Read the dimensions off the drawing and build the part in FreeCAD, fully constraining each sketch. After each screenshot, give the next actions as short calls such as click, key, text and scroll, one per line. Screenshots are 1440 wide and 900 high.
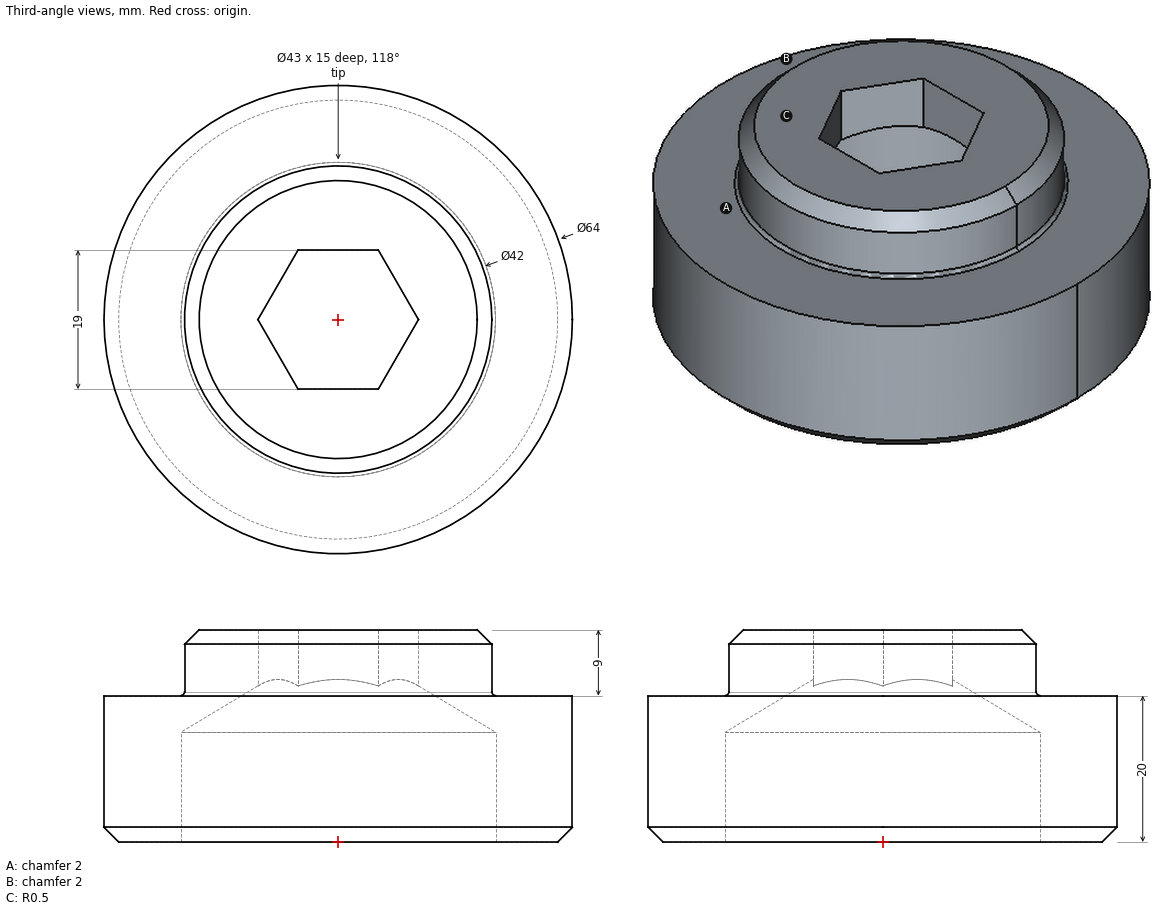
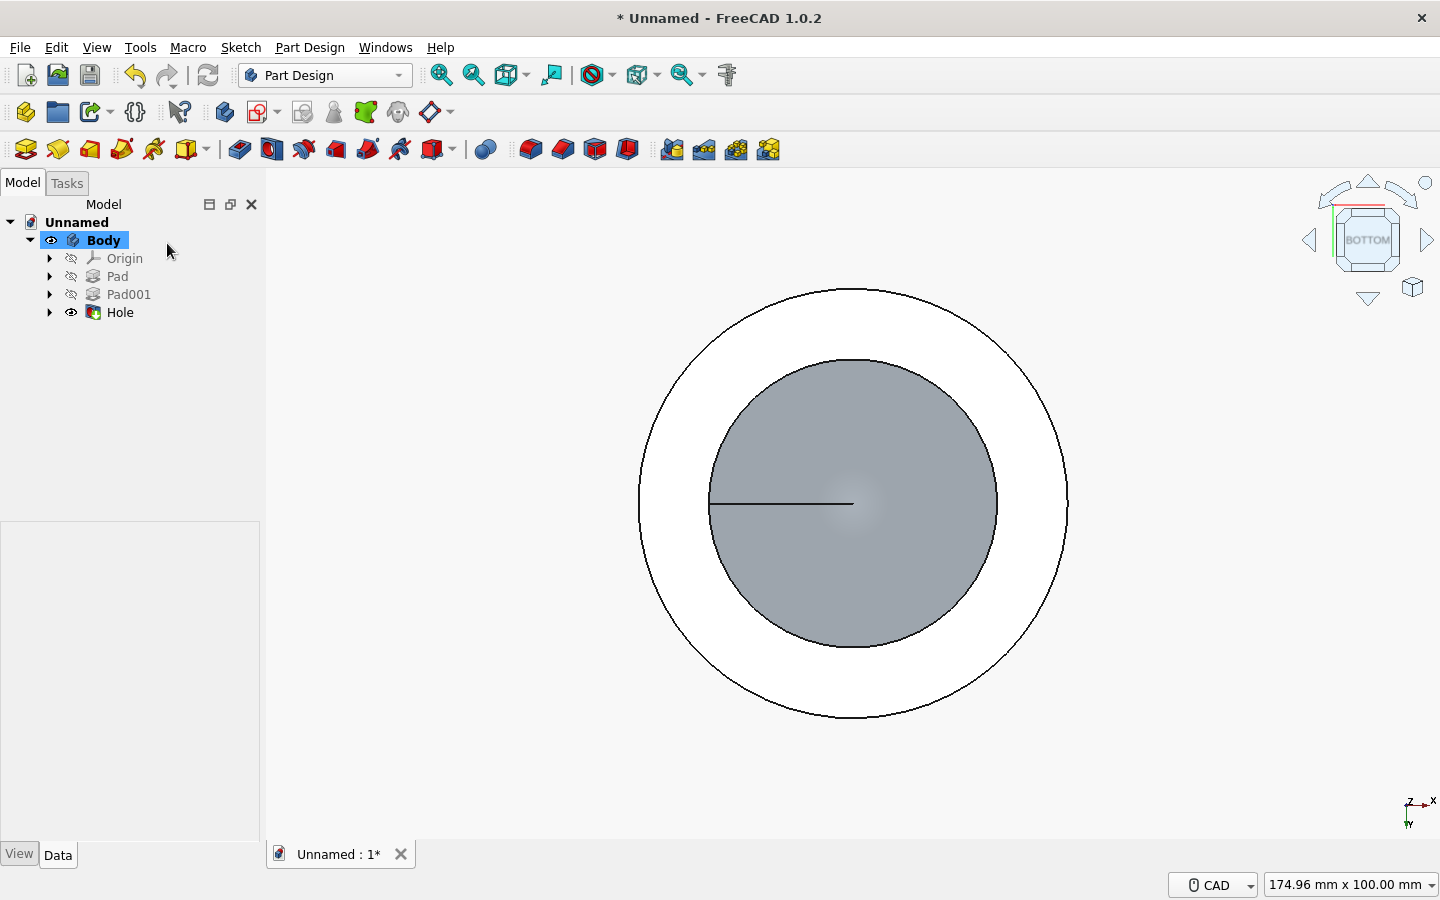
key(0)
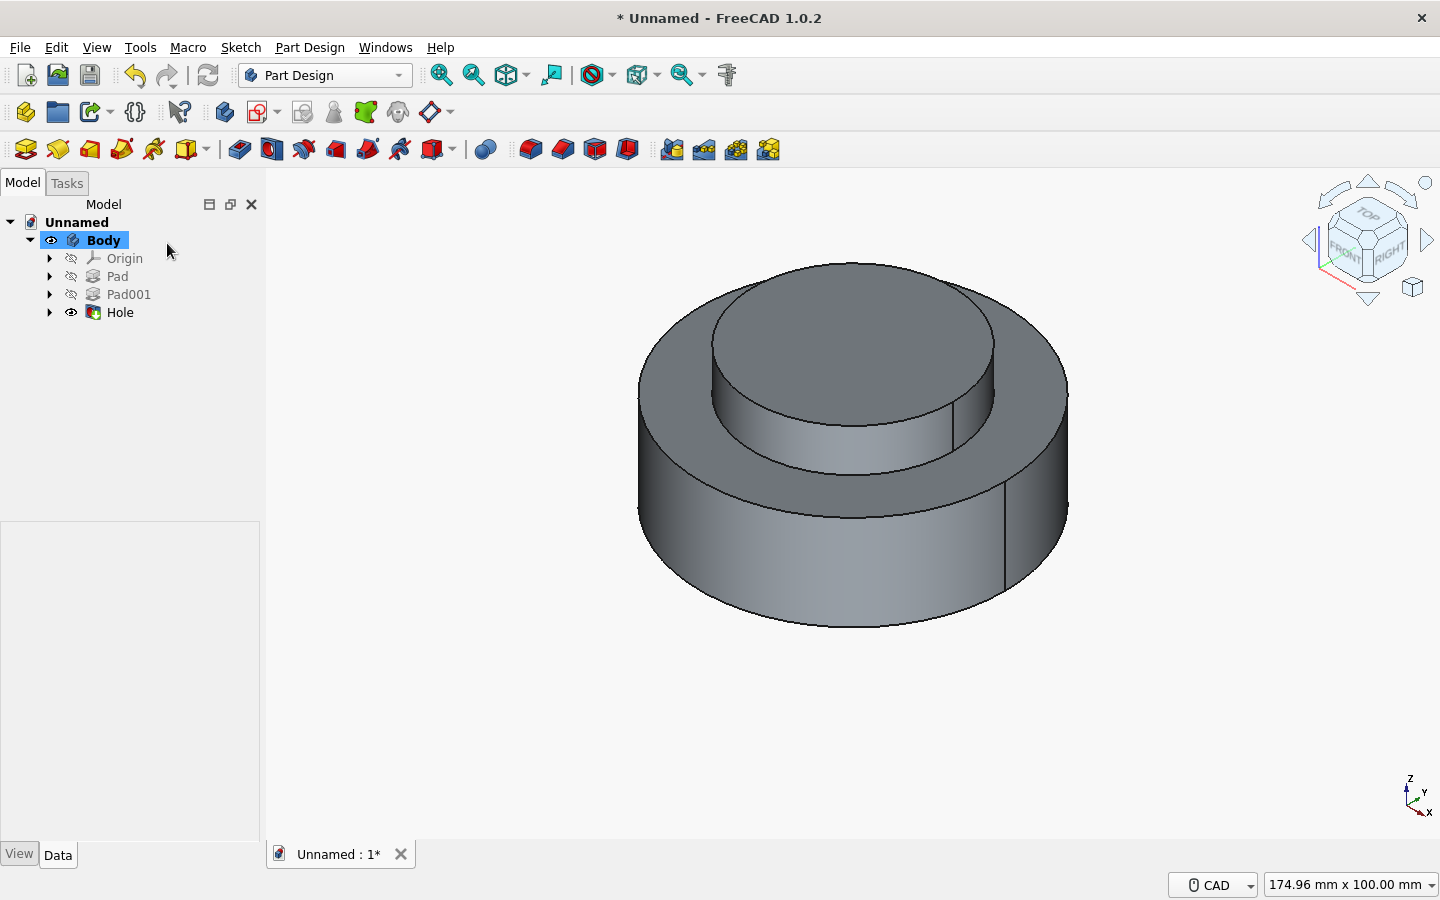
click(853, 344)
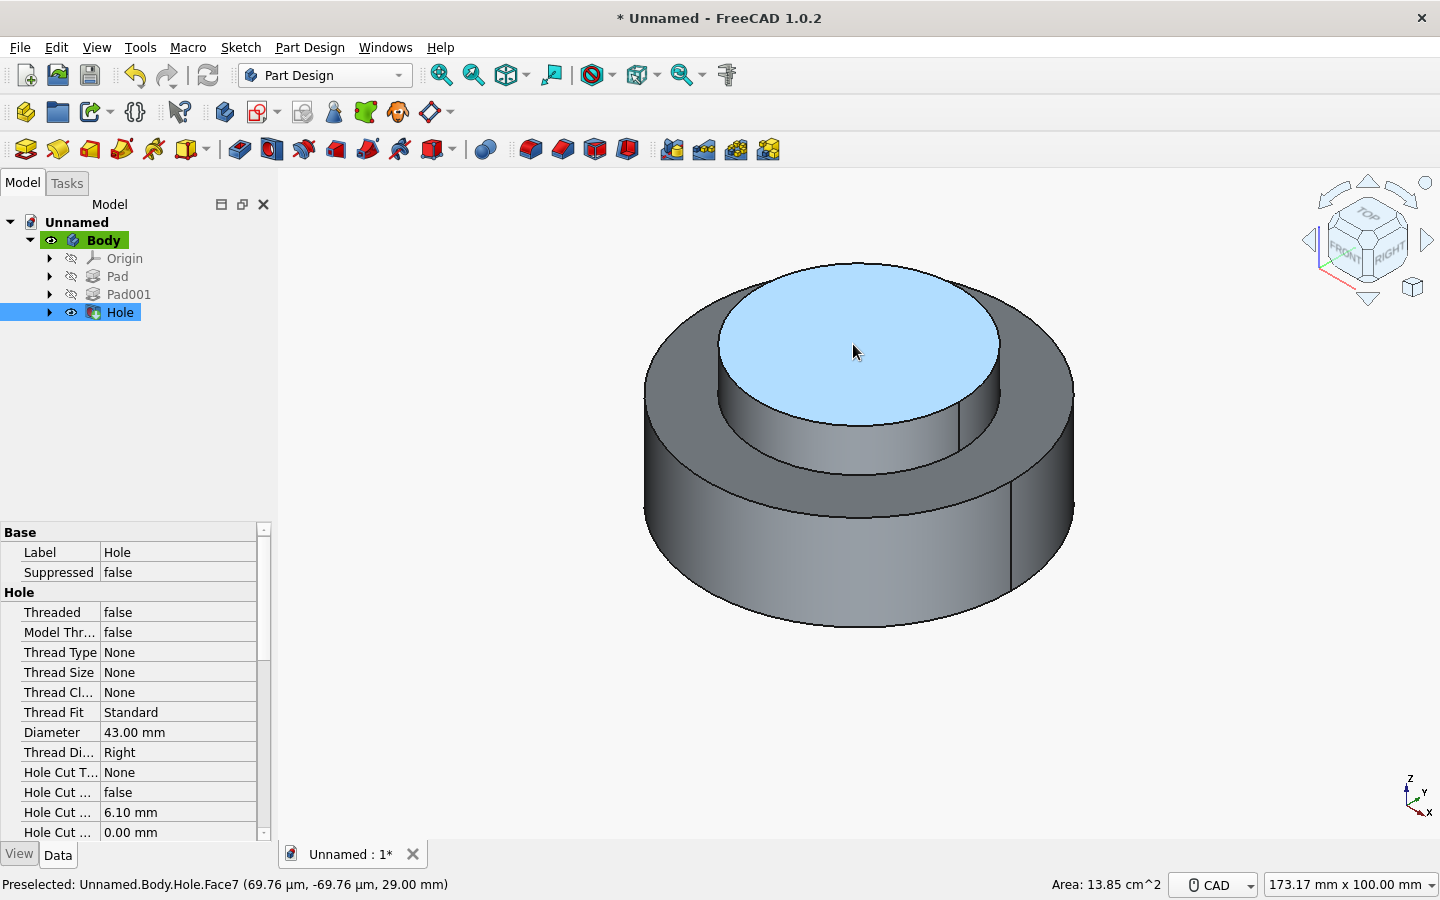
click(258, 112)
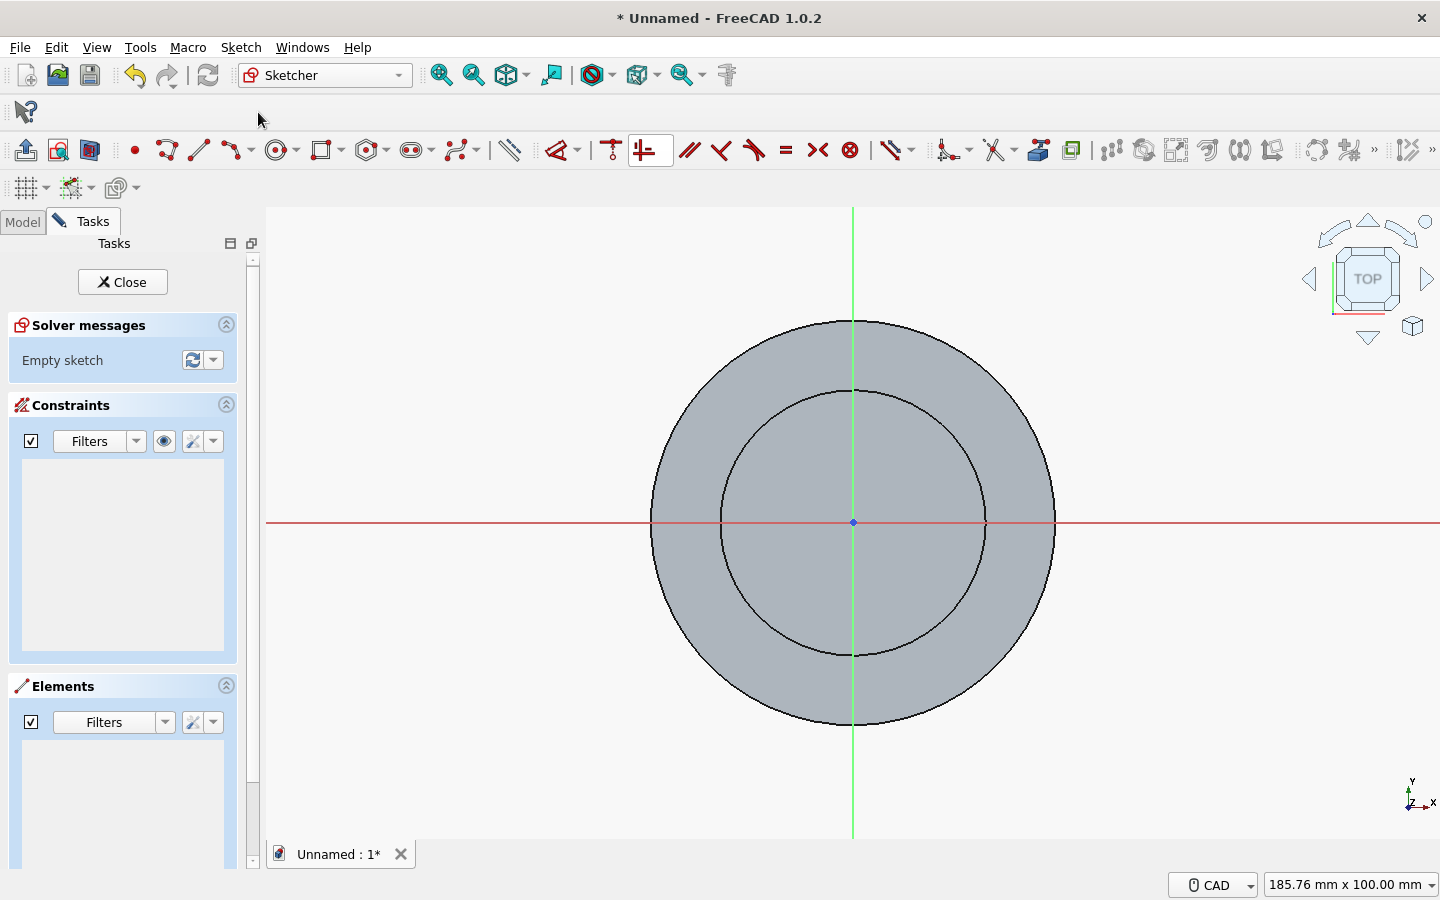
scroll(883, 523, up, 6)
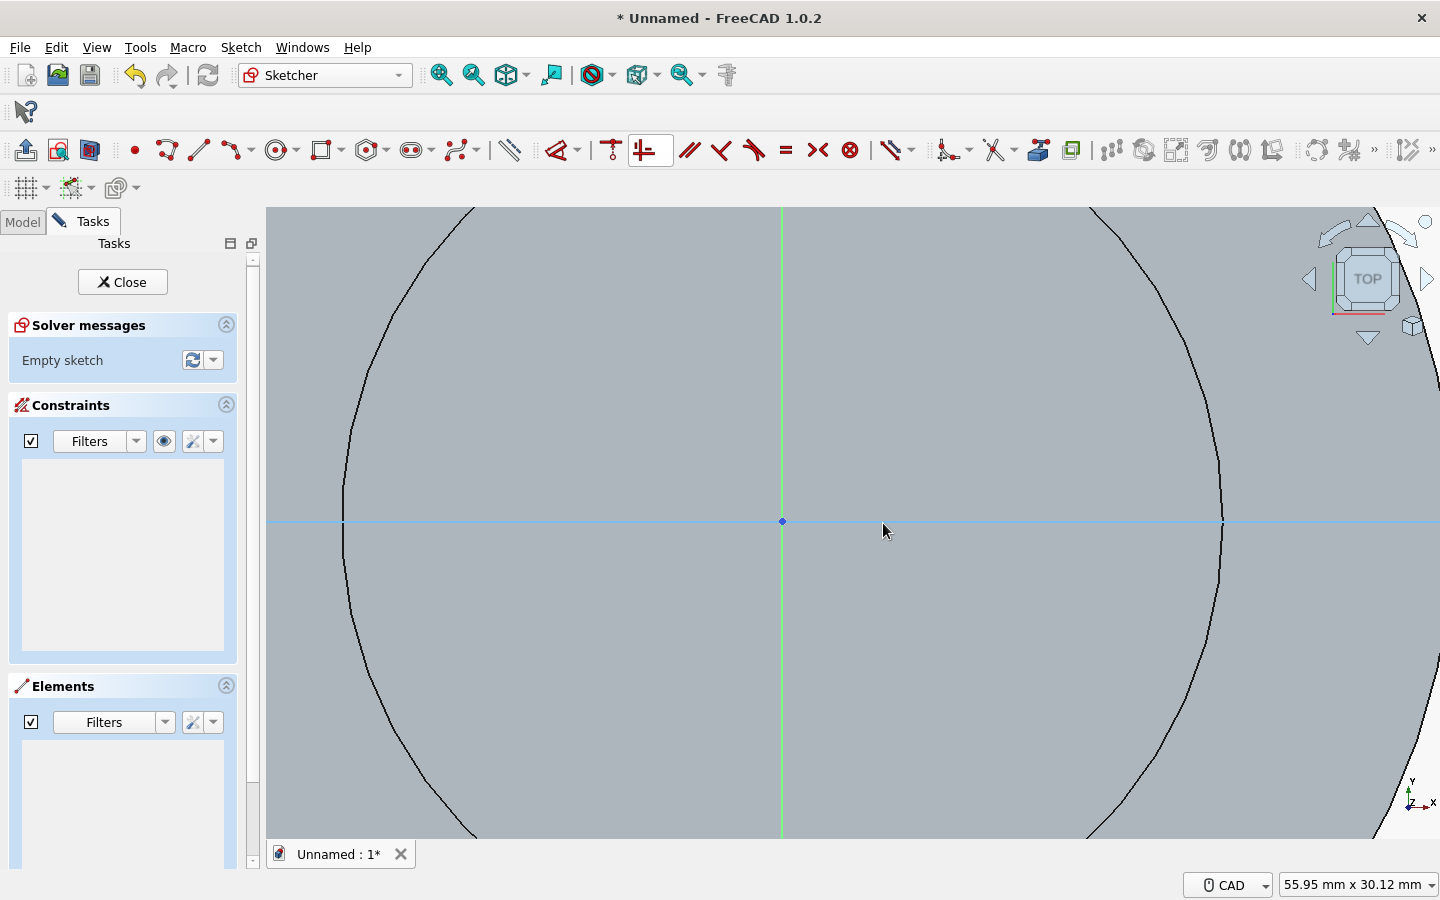
click(366, 150)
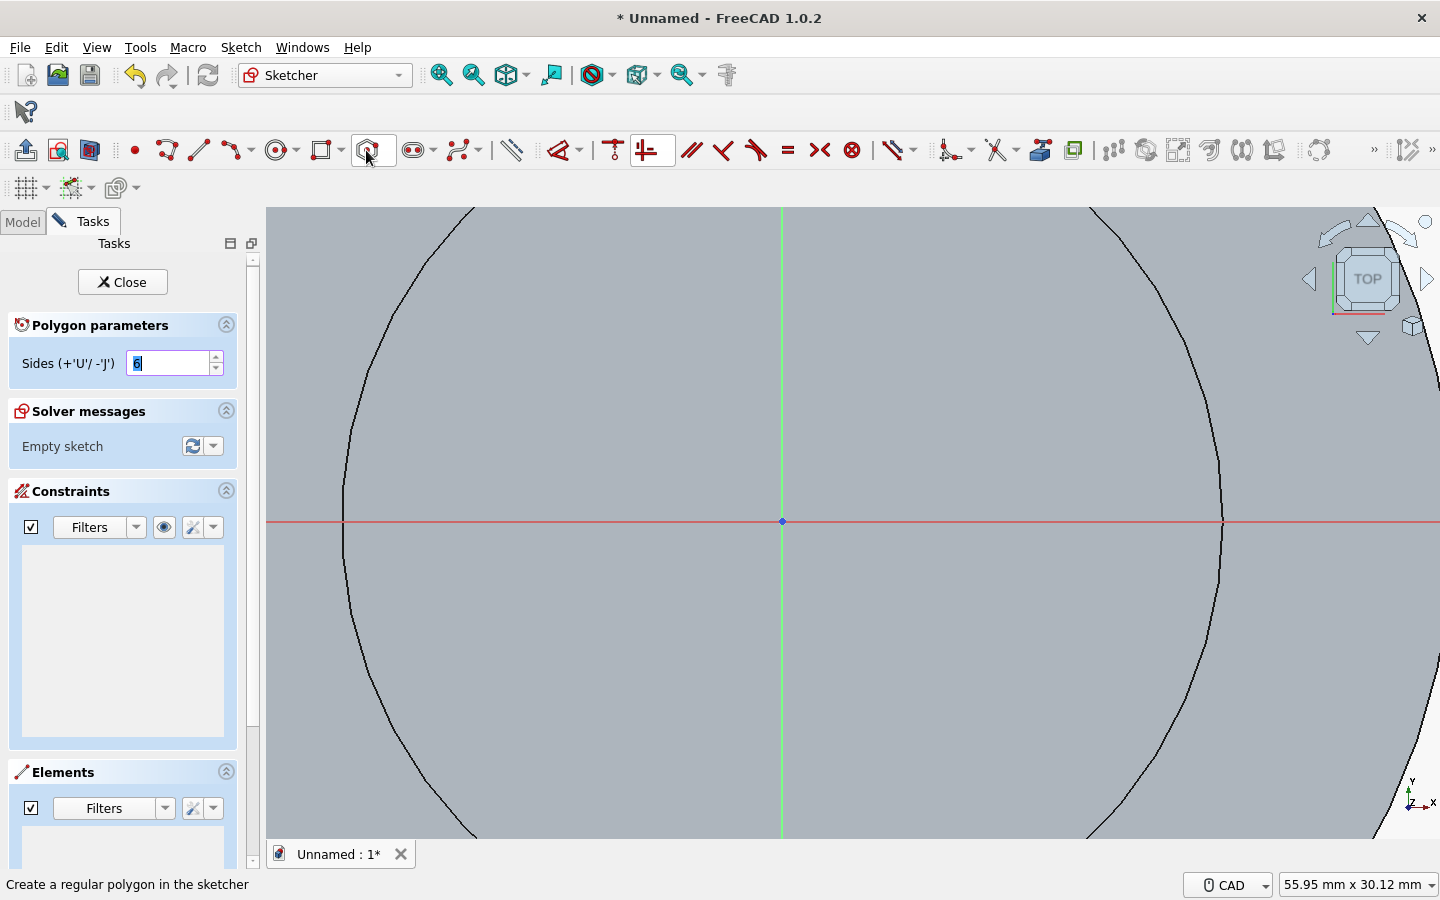
click(782, 522)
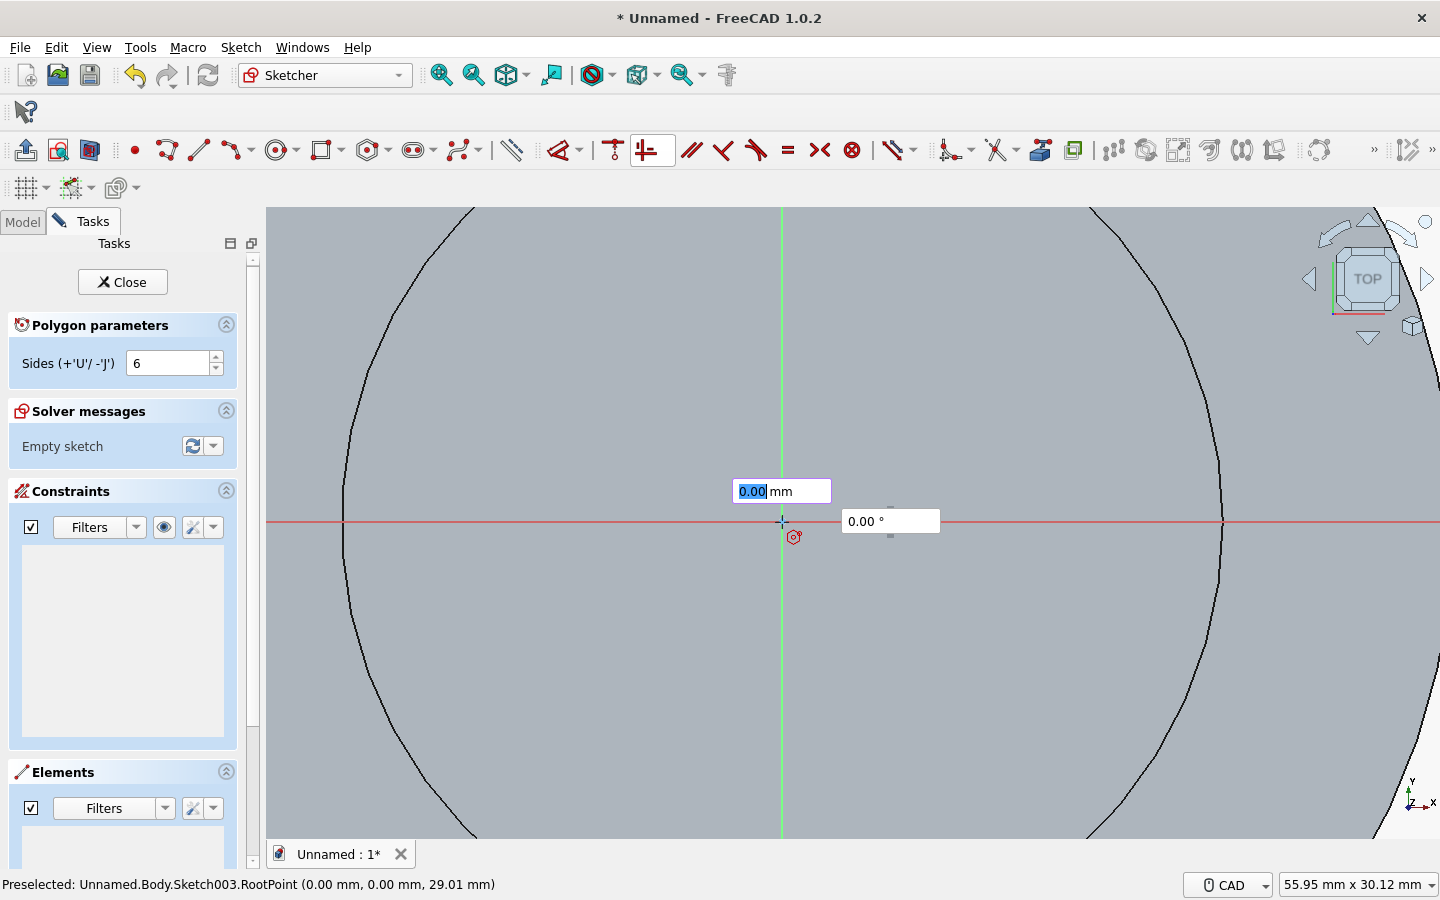
click(1012, 522)
key(Escape)